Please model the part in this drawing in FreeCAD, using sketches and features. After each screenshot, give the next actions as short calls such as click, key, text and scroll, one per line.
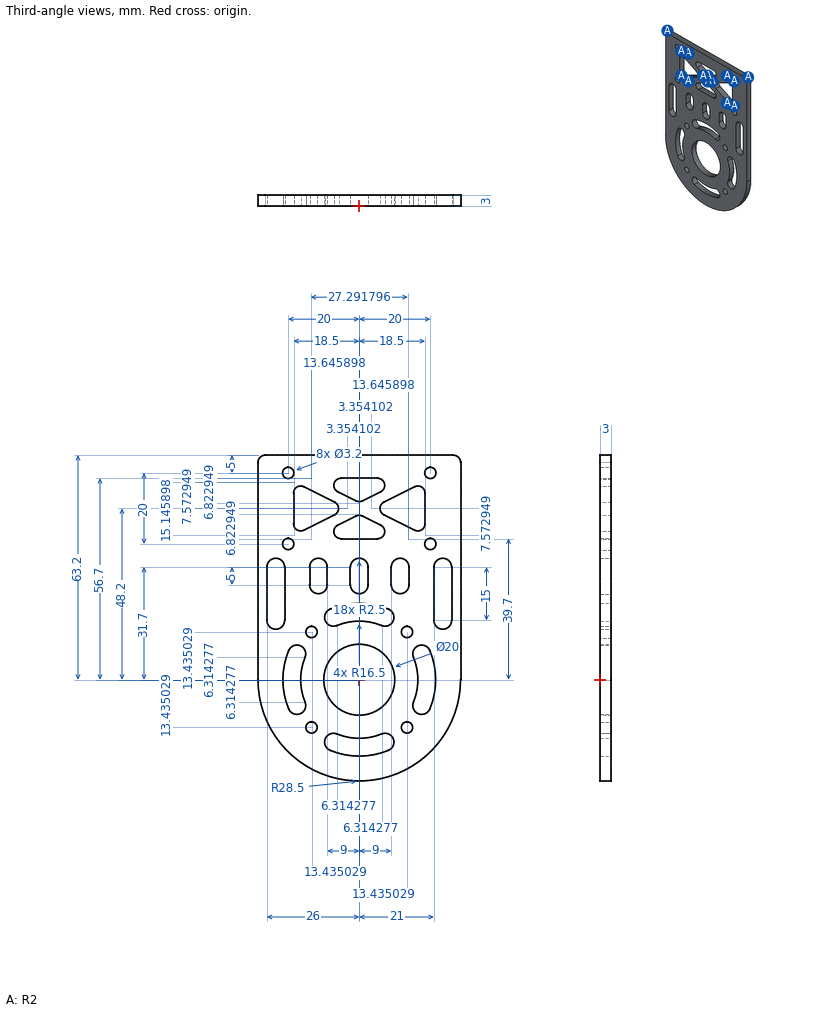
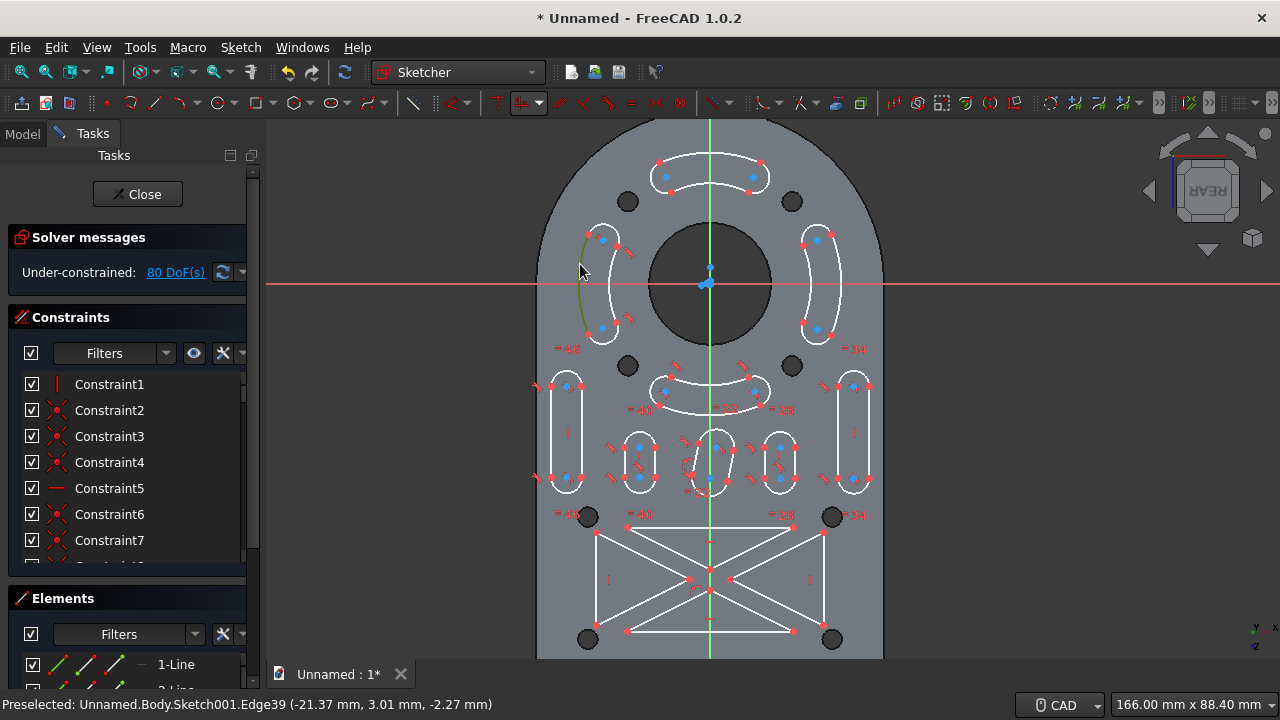
click(599, 344)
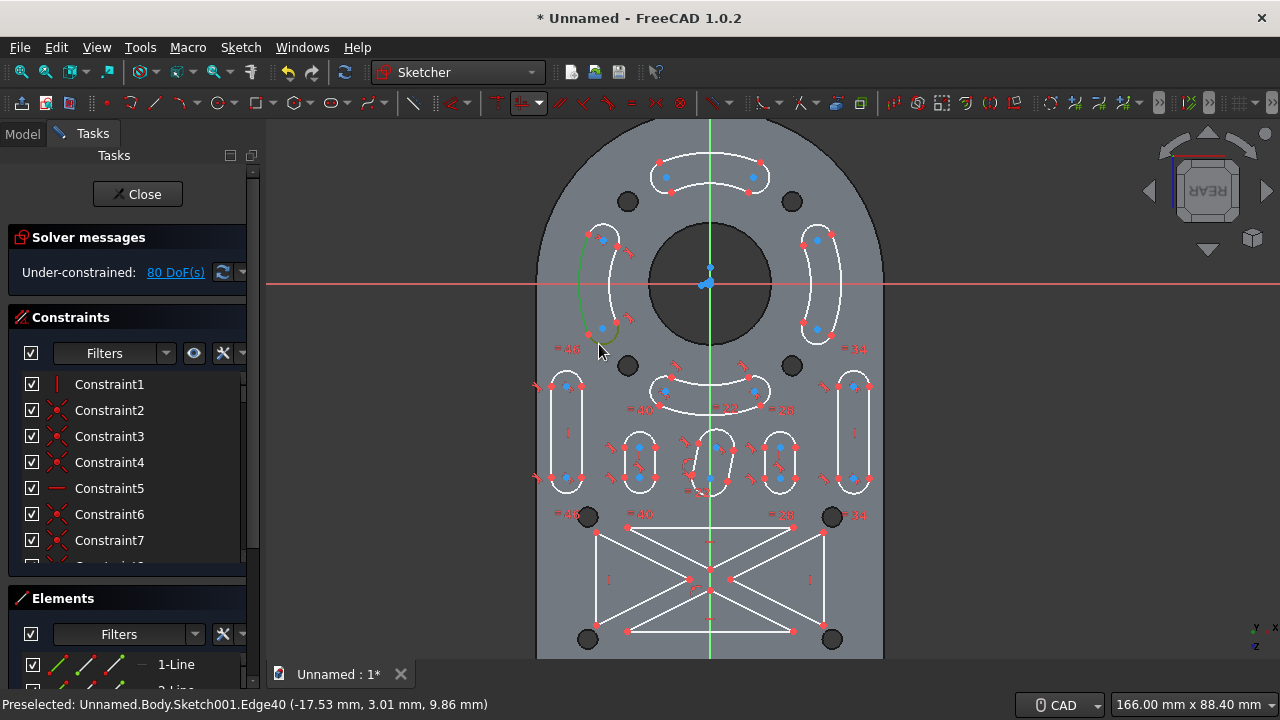
key(t)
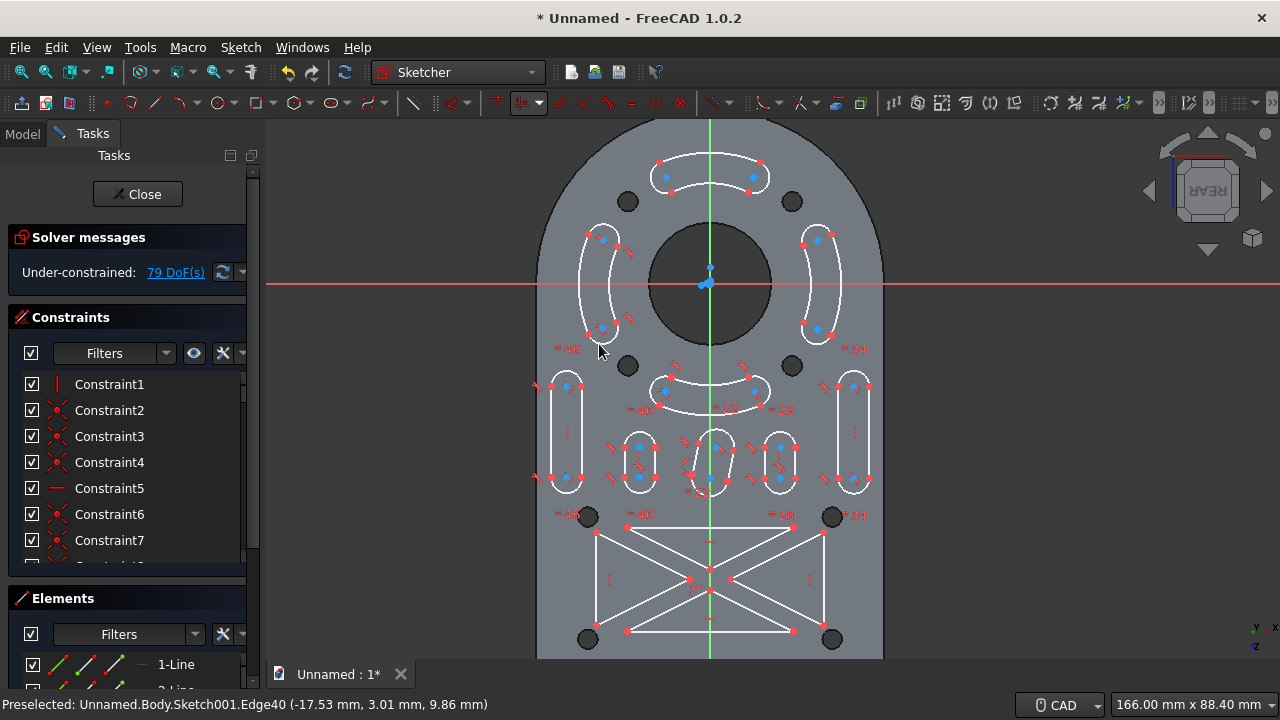
click(810, 300)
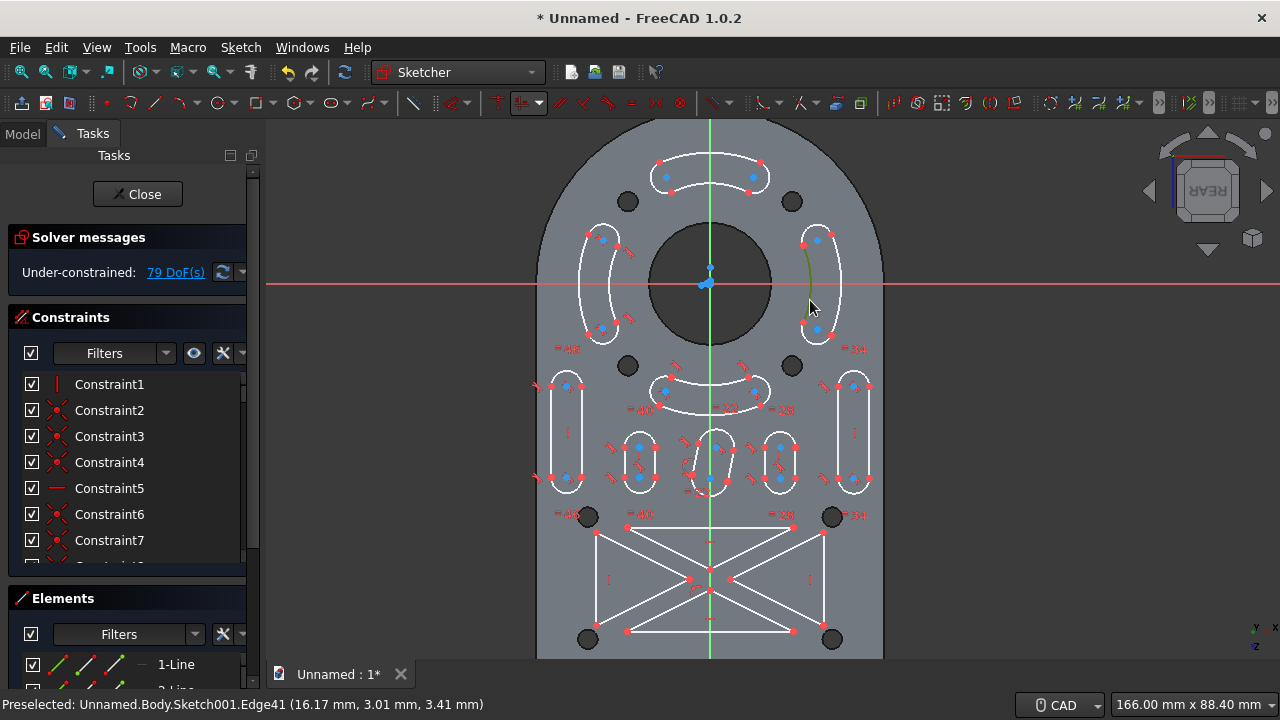
click(804, 337)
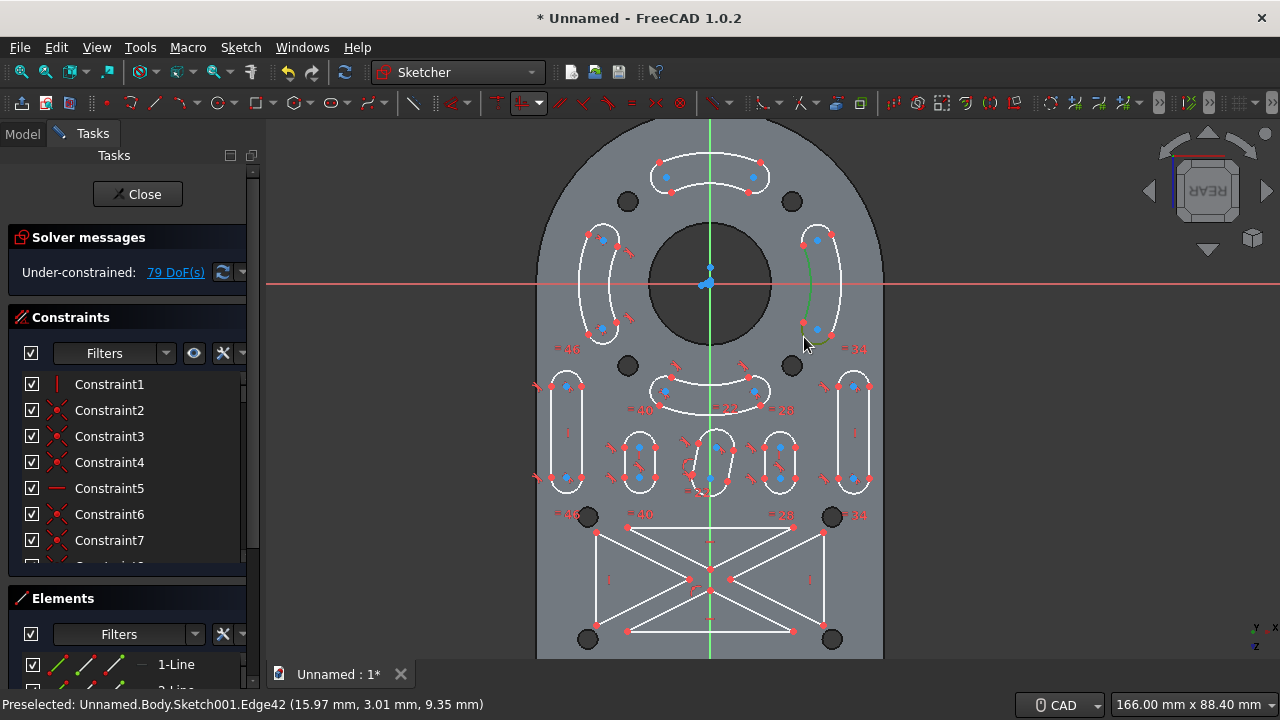
click(608, 104)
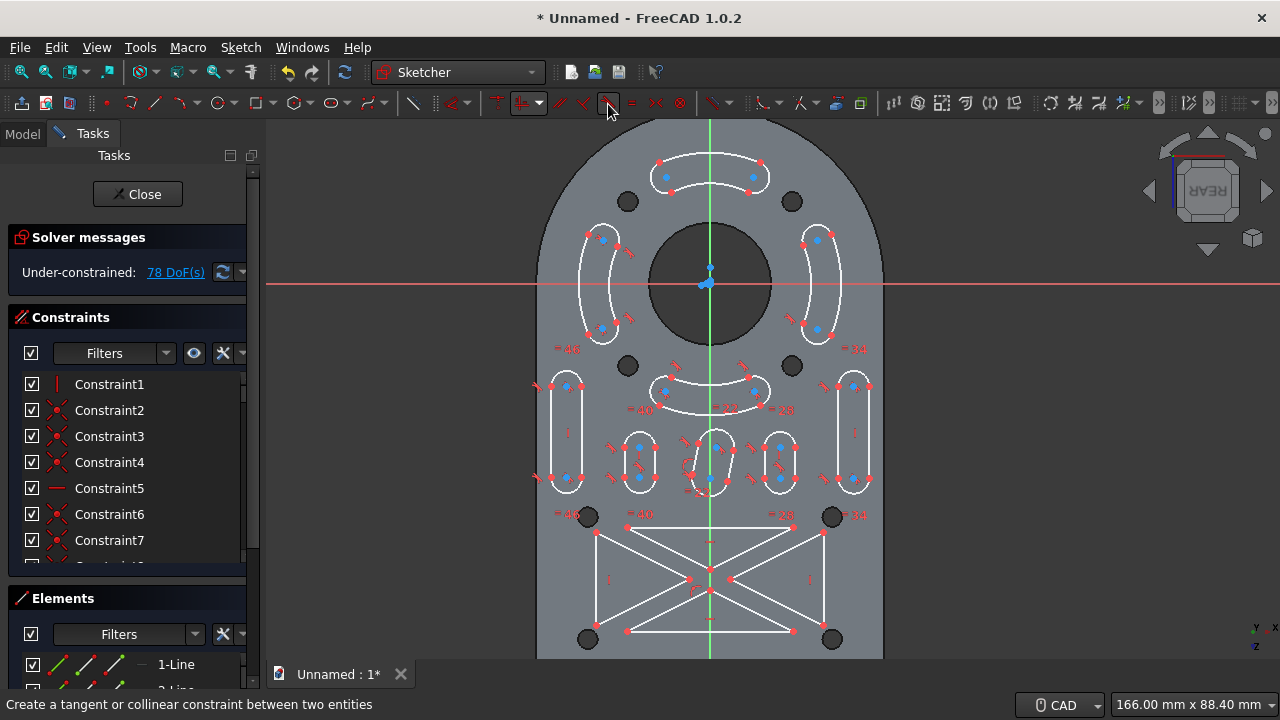
click(810, 300)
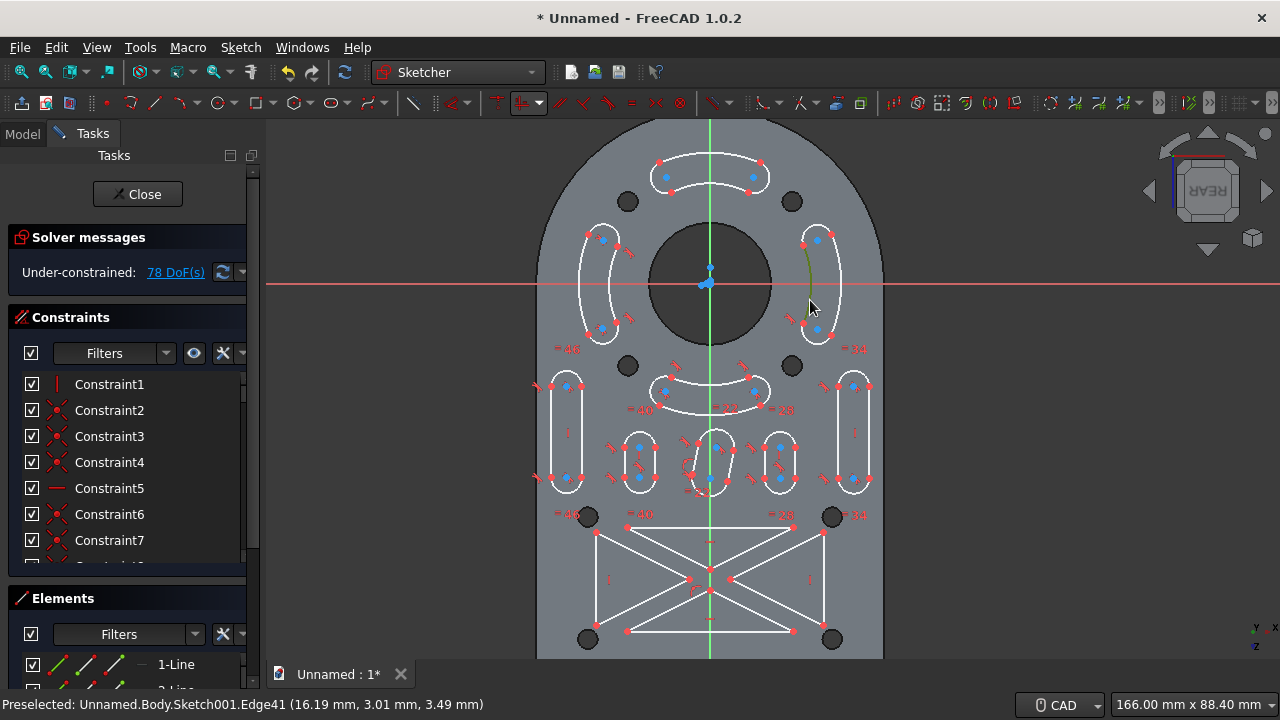
click(821, 225)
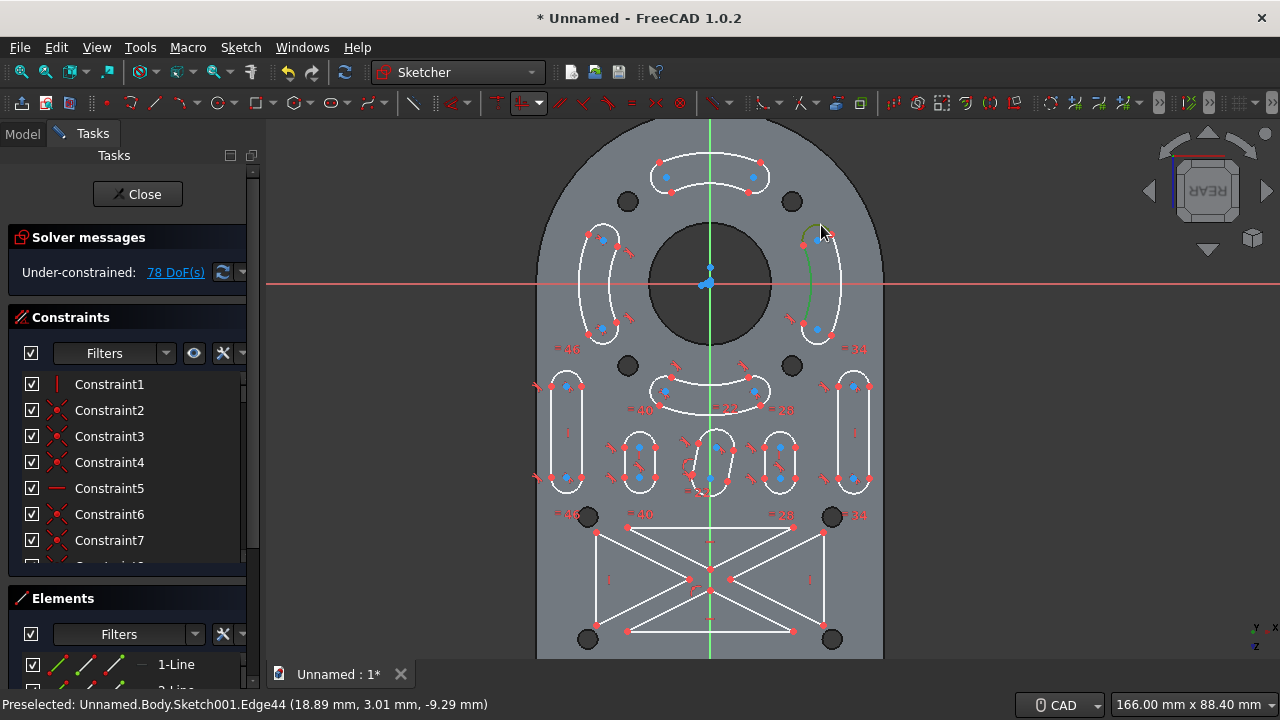
key(t)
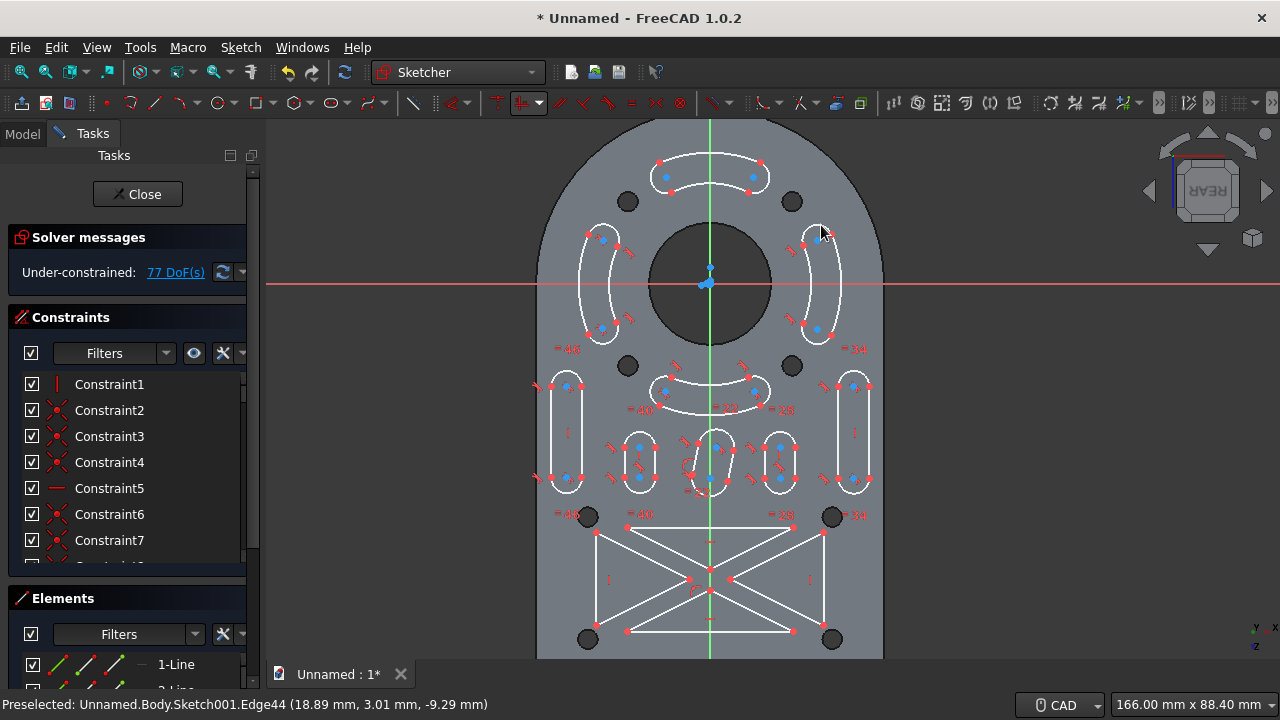
click(804, 337)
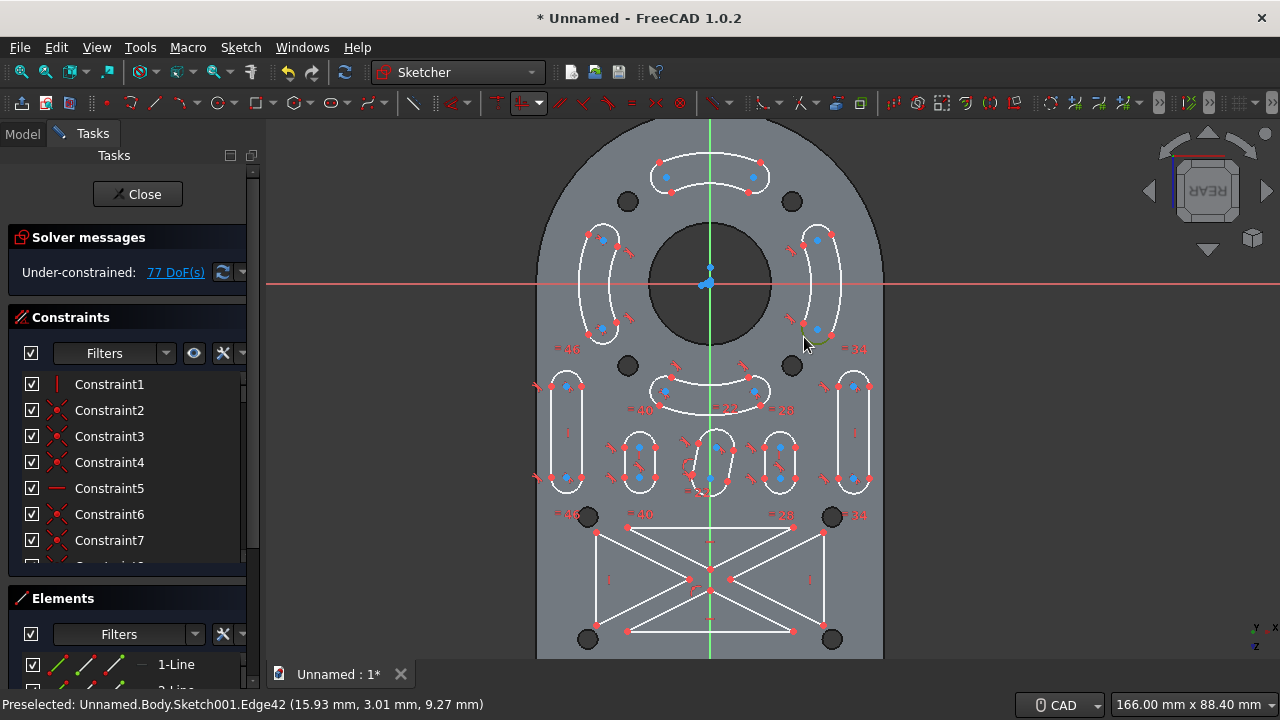
click(839, 305)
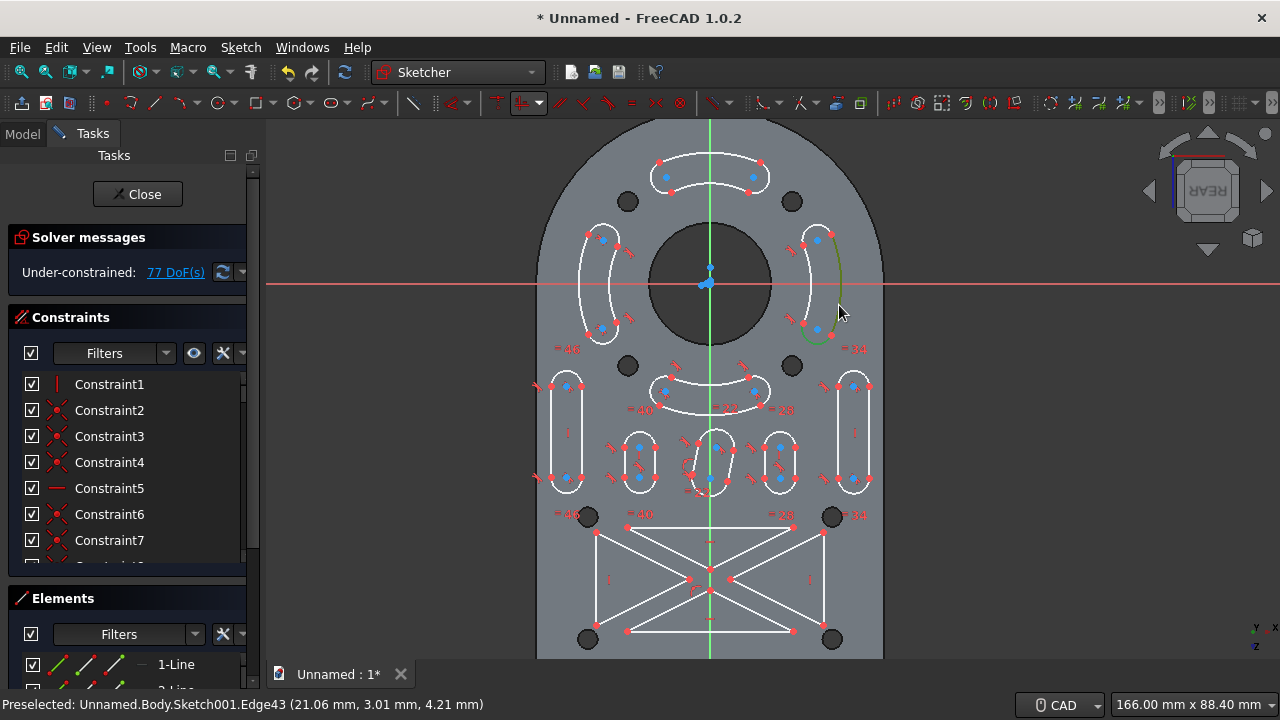
key(t)